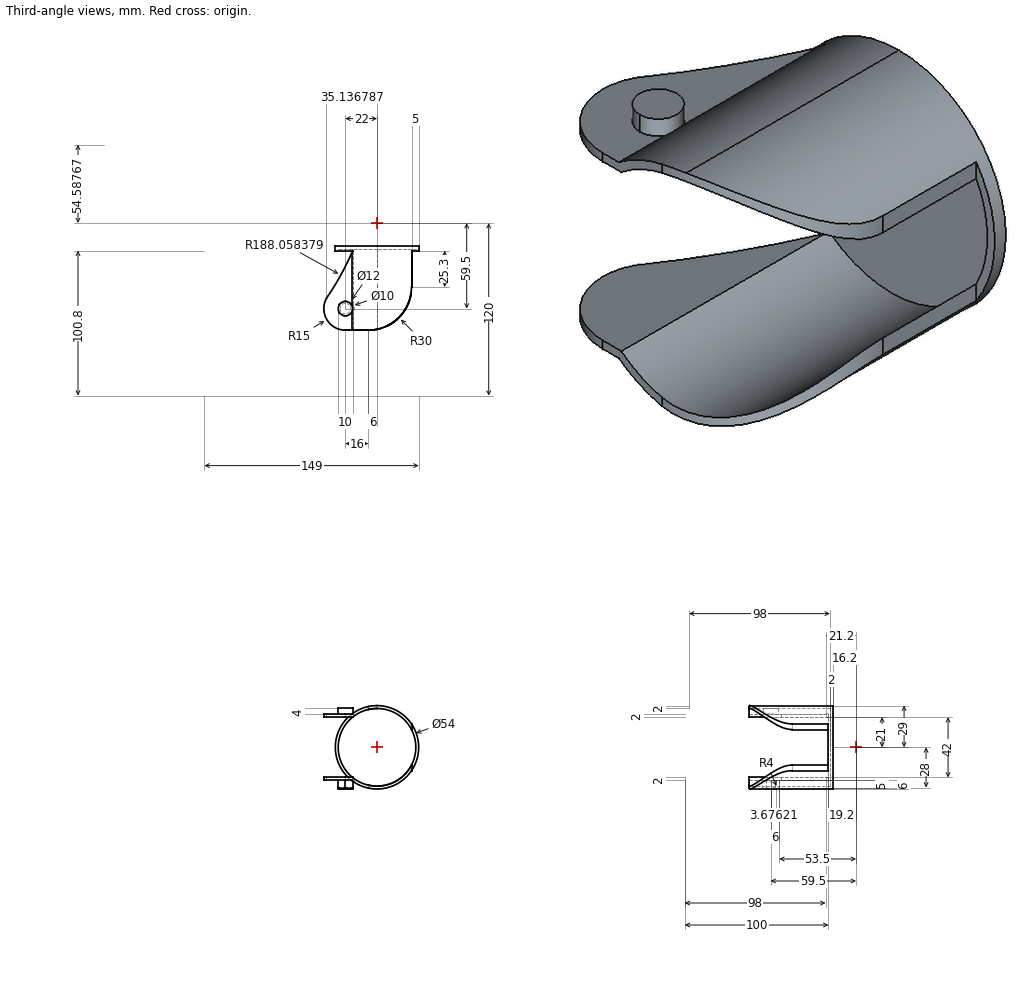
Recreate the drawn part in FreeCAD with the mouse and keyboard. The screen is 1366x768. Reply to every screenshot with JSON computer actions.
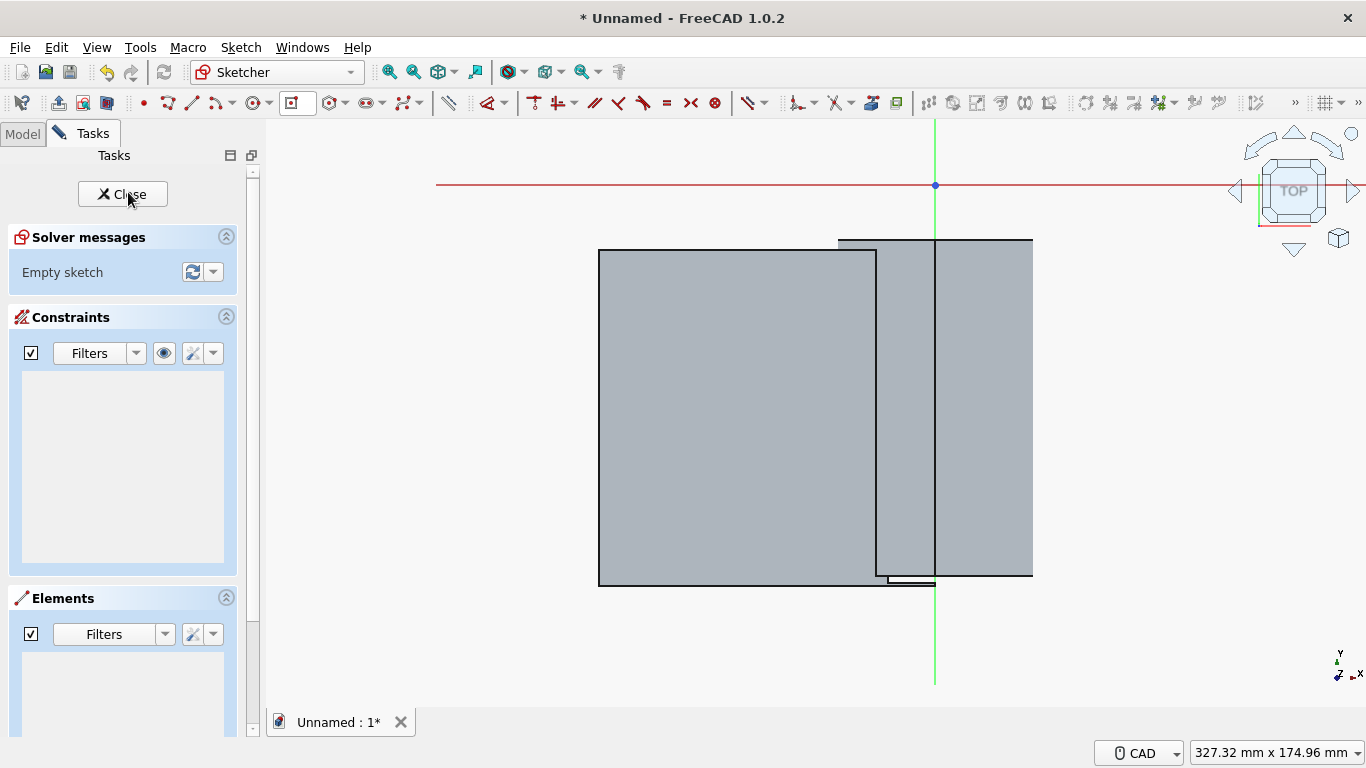
{"action": "left_click", "coordinate": [108, 104]}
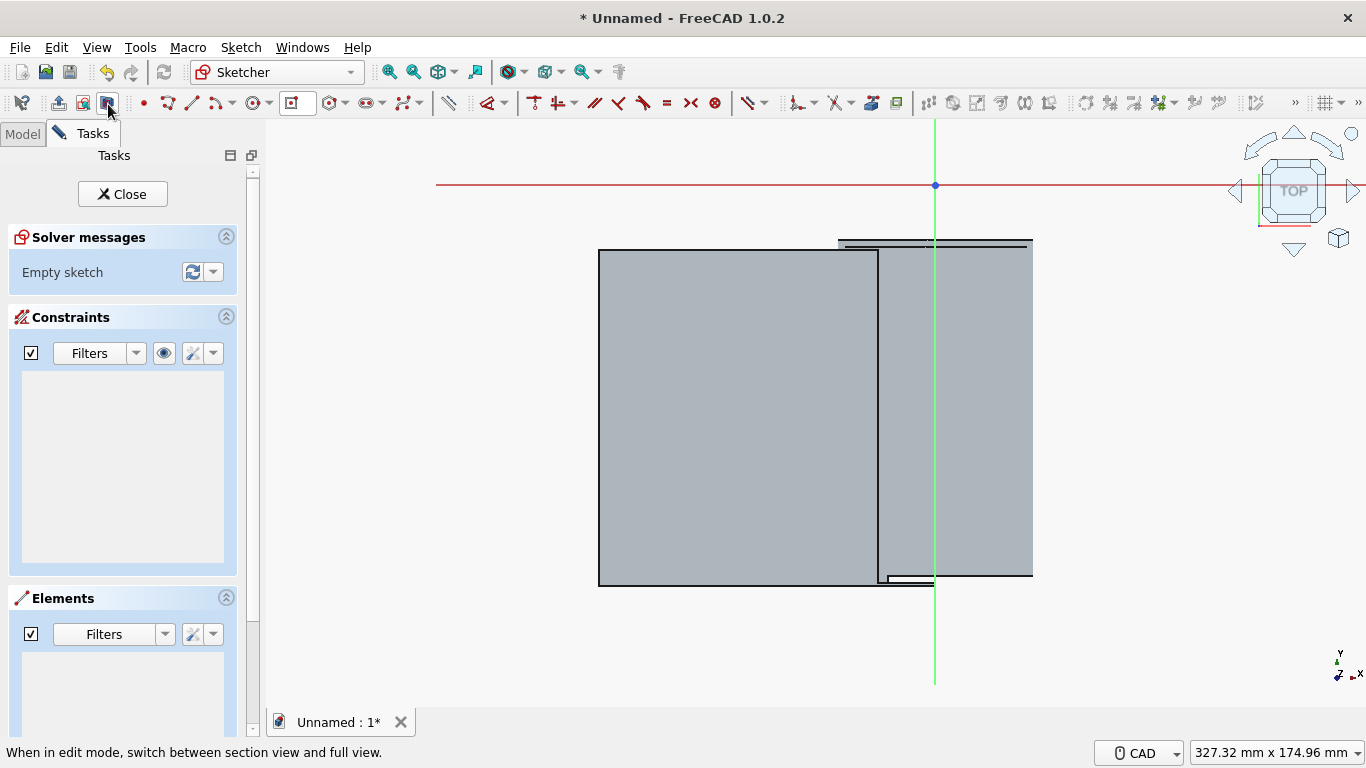
{"action": "left_click", "coordinate": [192, 104]}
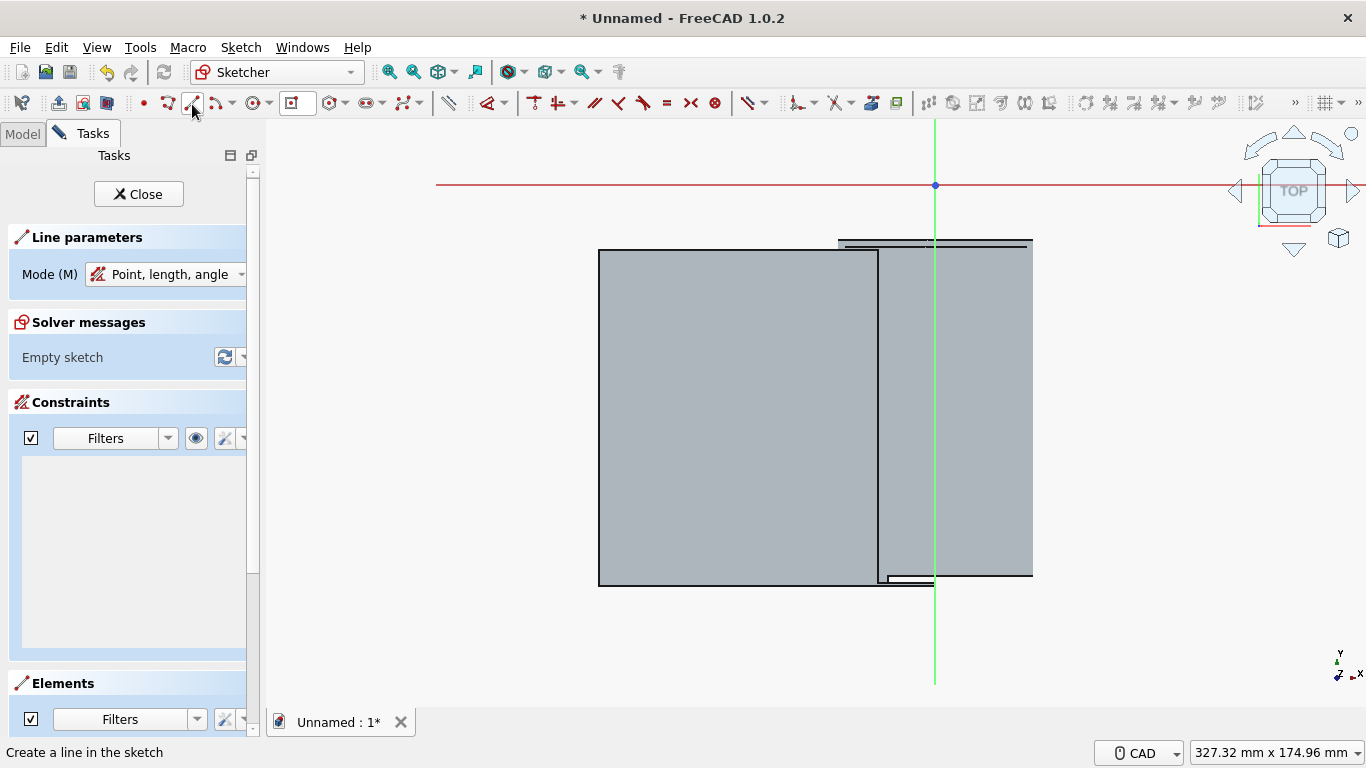
{"action": "left_click", "coordinate": [915, 436]}
{"action": "left_click", "coordinate": [861, 436]}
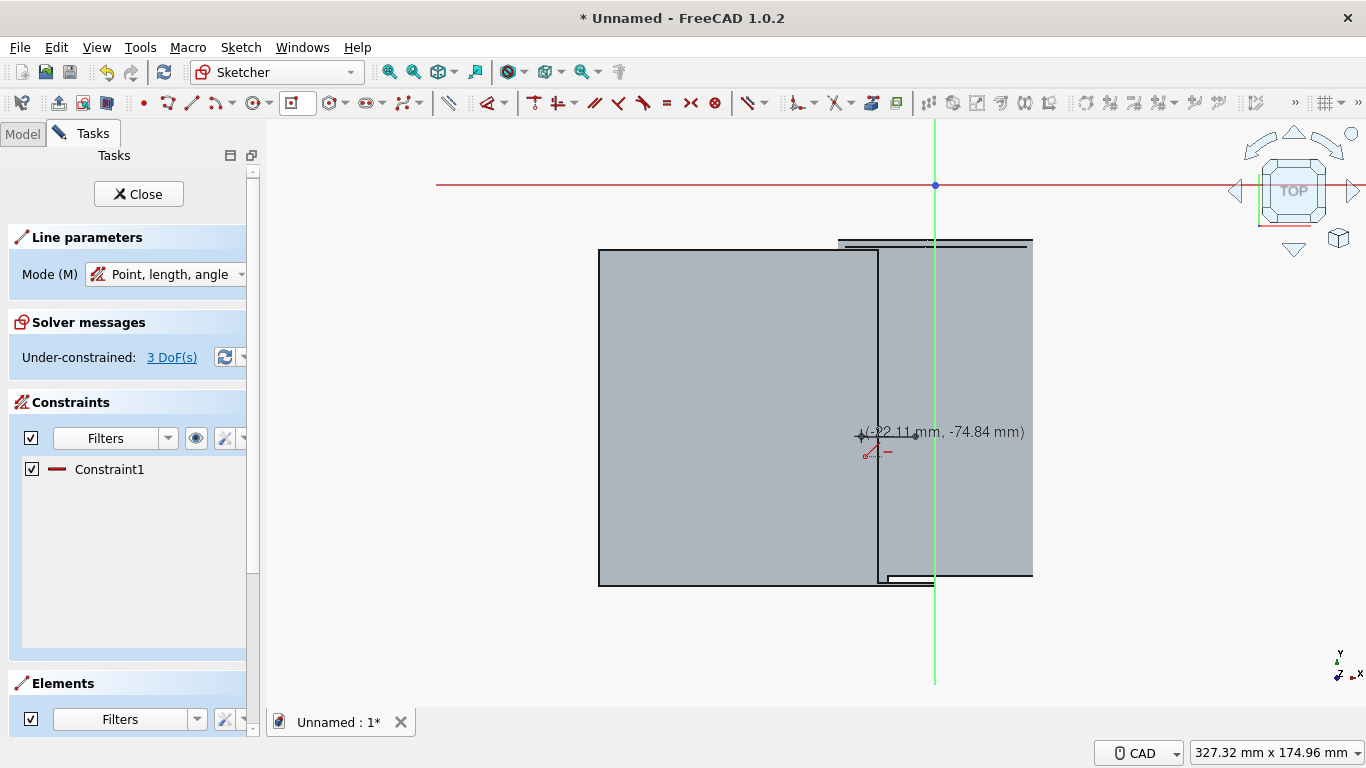
{"action": "left_click", "coordinate": [168, 104]}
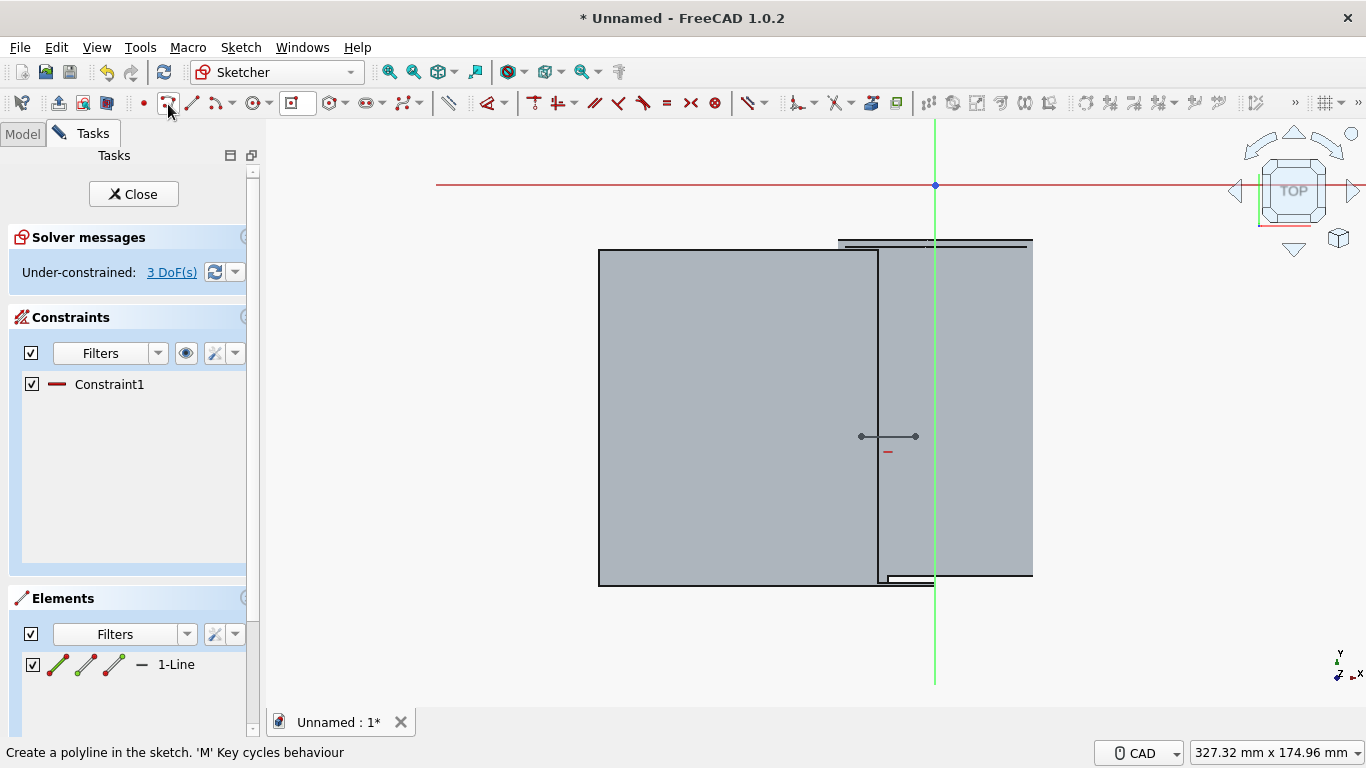
{"action": "left_click", "coordinate": [878, 250]}
{"action": "left_click", "coordinate": [532, 250]}
{"action": "left_click", "coordinate": [532, 589]}
{"action": "left_click", "coordinate": [1033, 589]}
{"action": "left_click", "coordinate": [1033, 250]}
{"action": "left_click", "coordinate": [1016, 250]}
{"action": "left_click", "coordinate": [1016, 335]}
{"action": "right_click", "coordinate": [1016, 335]}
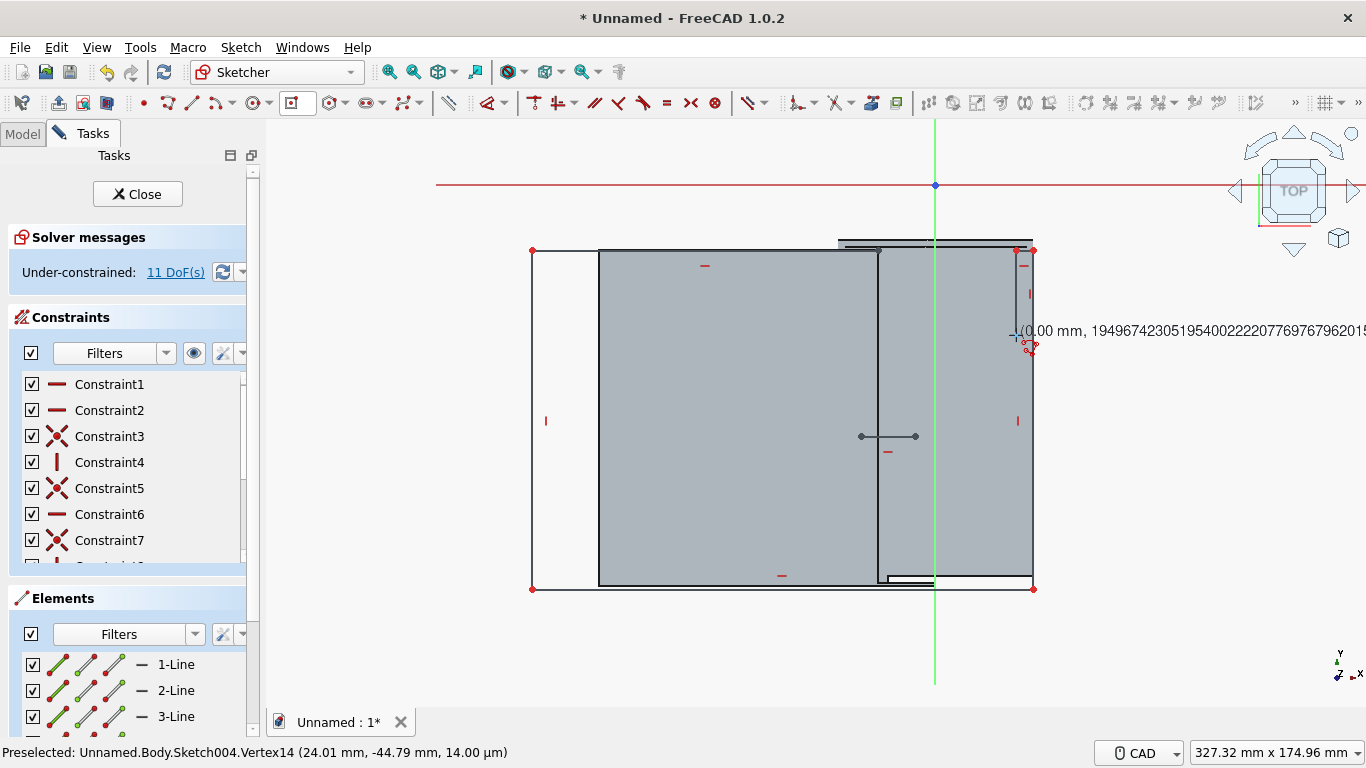
{"action": "key", "text": "g 3 a"}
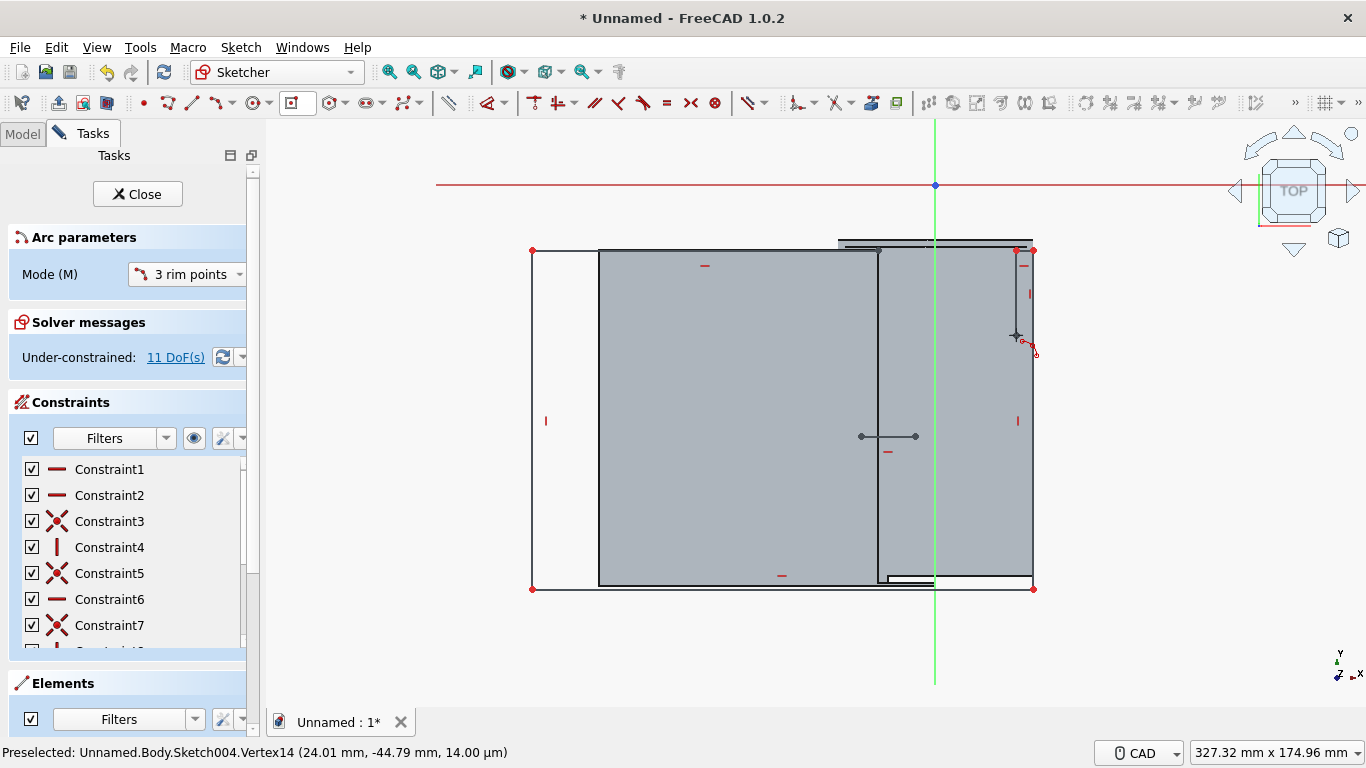
{"action": "left_click", "coordinate": [861, 437]}
{"action": "left_click", "coordinate": [817, 361]}
{"action": "left_click", "coordinate": [818, 411]}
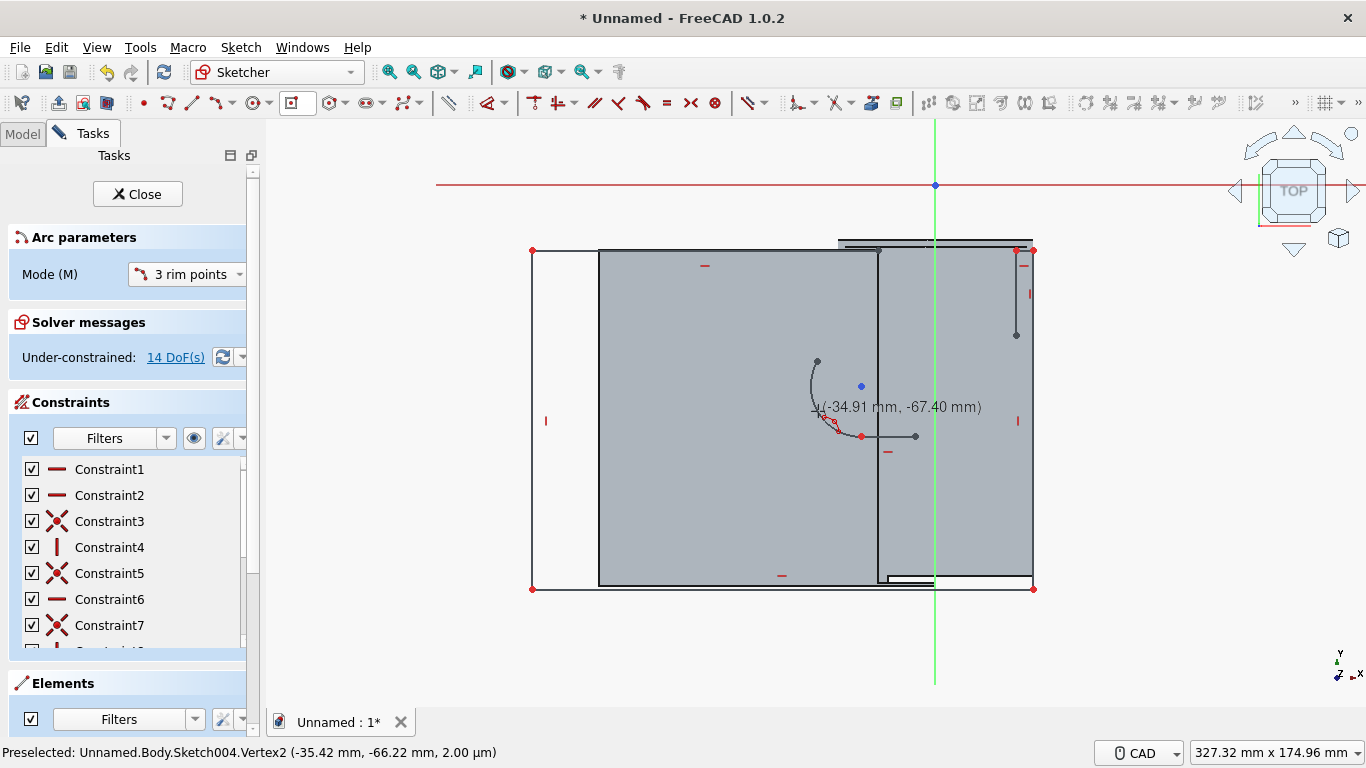
{"action": "left_click", "coordinate": [817, 362]}
{"action": "left_click", "coordinate": [878, 251]}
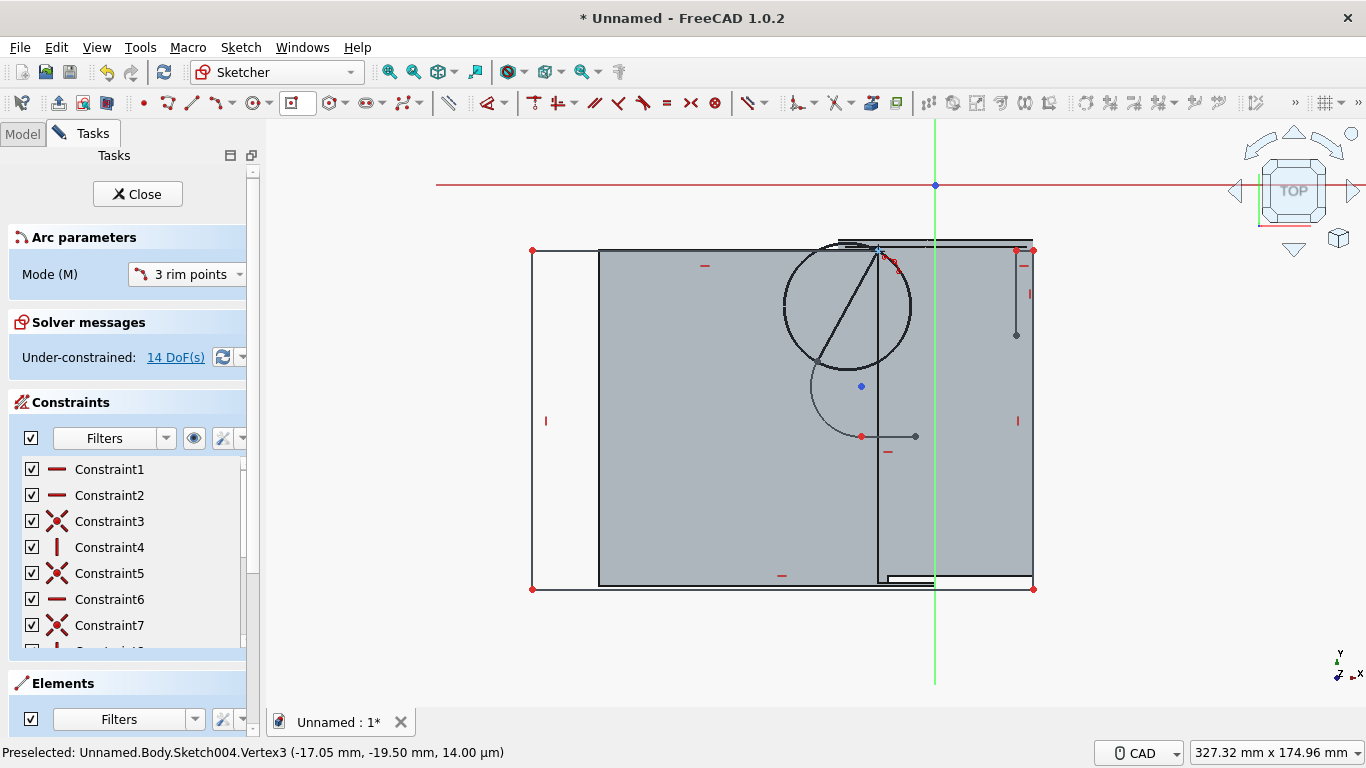
{"action": "scroll", "coordinate": [851, 307], "scroll_direction": "up", "scroll_amount": 9}